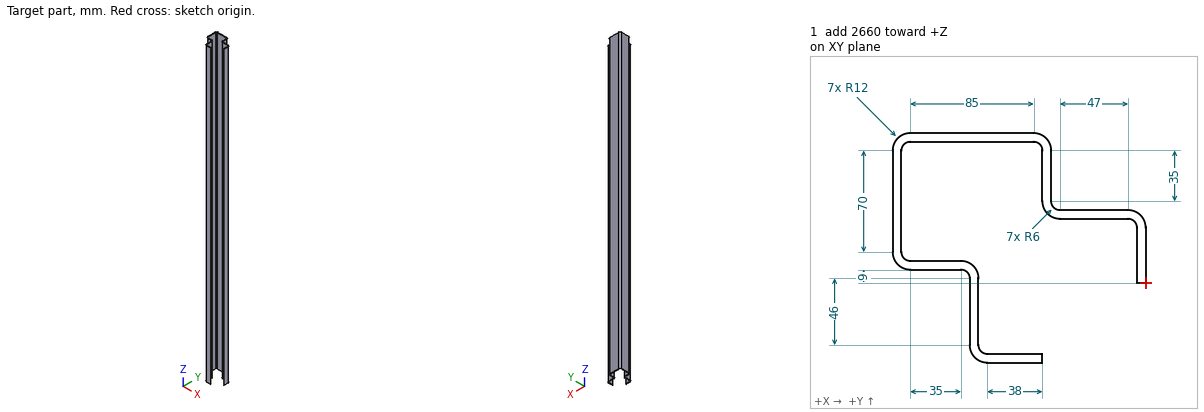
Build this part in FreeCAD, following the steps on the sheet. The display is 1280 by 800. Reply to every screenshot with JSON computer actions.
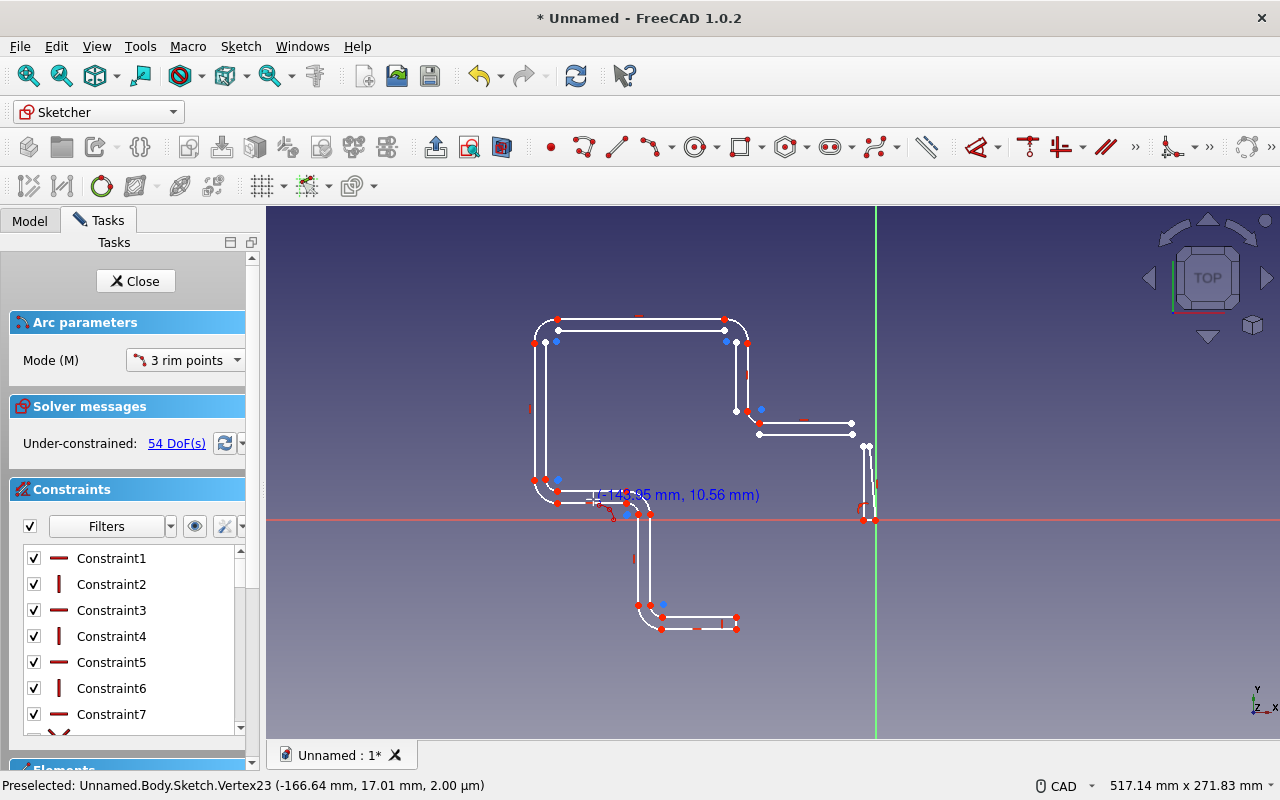
{"action": "scroll", "coordinate": [546, 342], "scroll_direction": "up", "scroll_amount": 2}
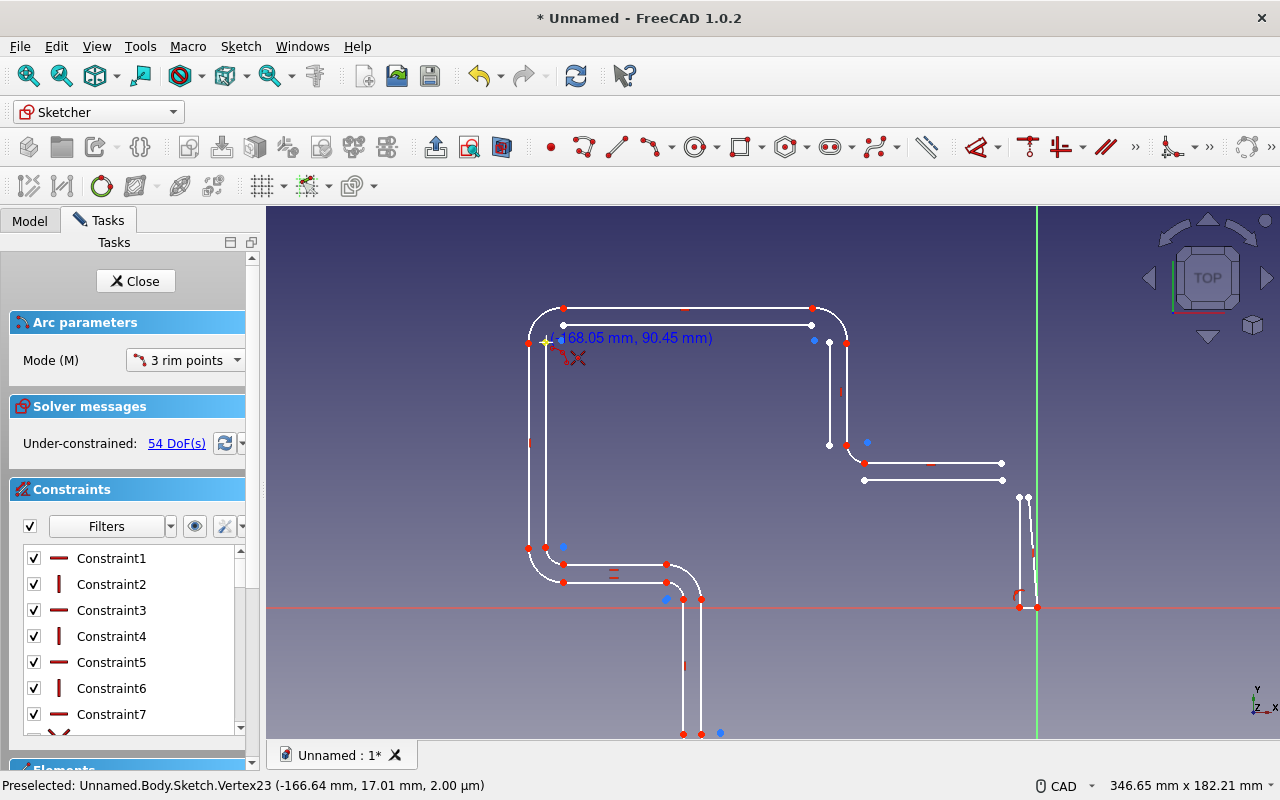
{"action": "left_click", "coordinate": [546, 342]}
{"action": "left_click", "coordinate": [564, 325]}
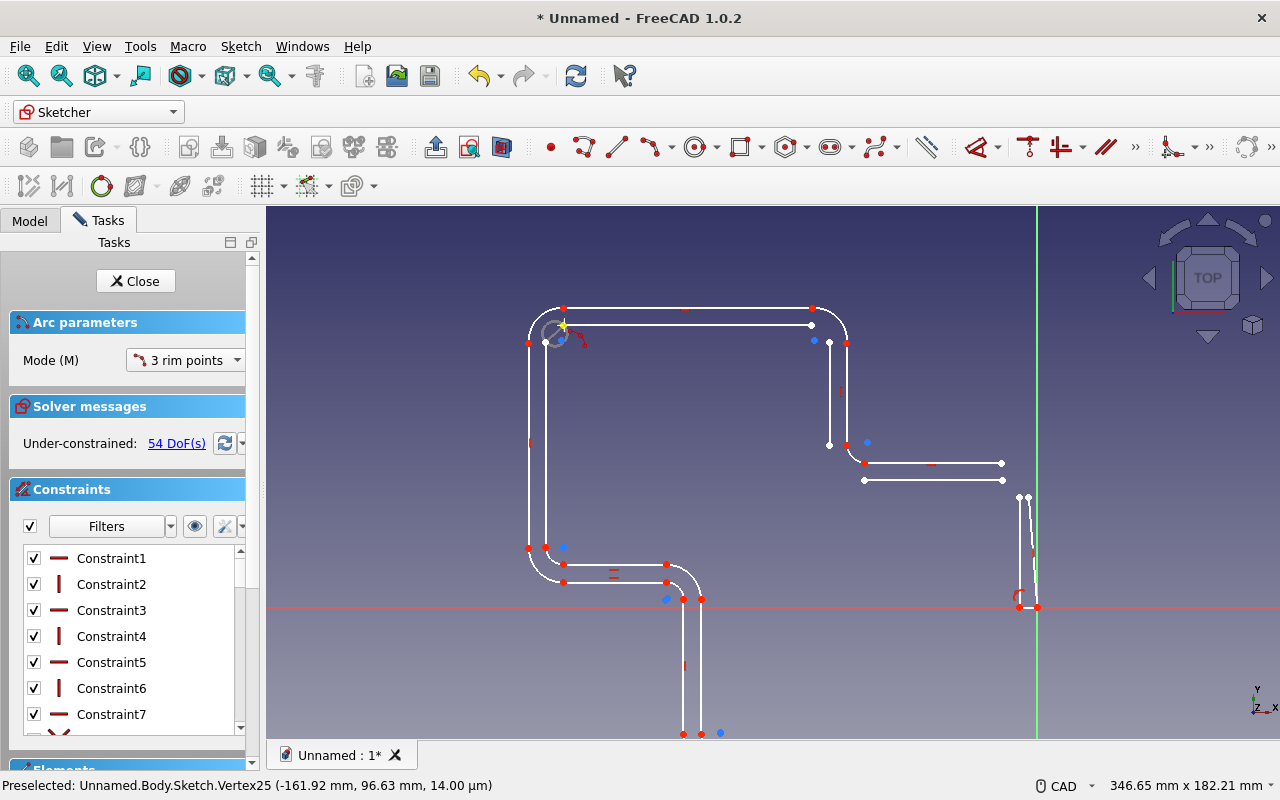
{"action": "scroll", "coordinate": [551, 329], "scroll_direction": "up", "scroll_amount": 6}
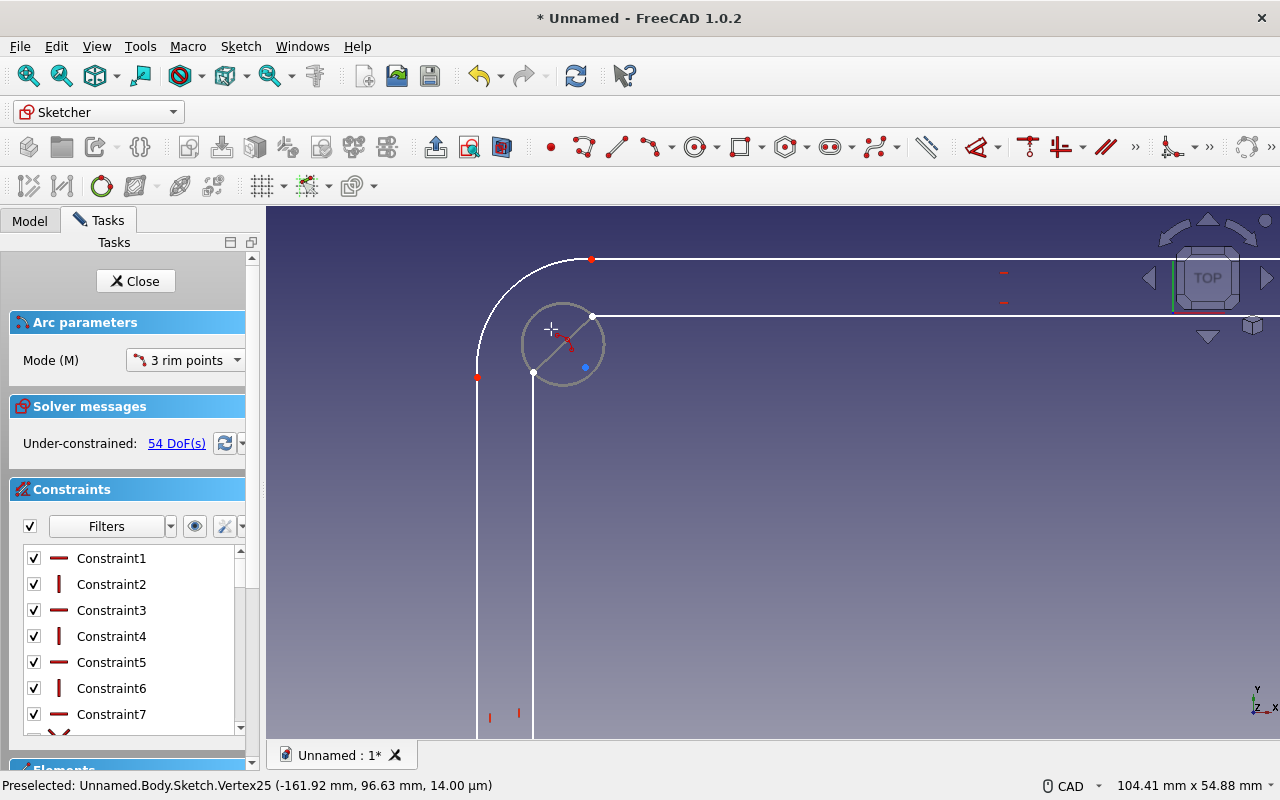
{"action": "left_click", "coordinate": [551, 330]}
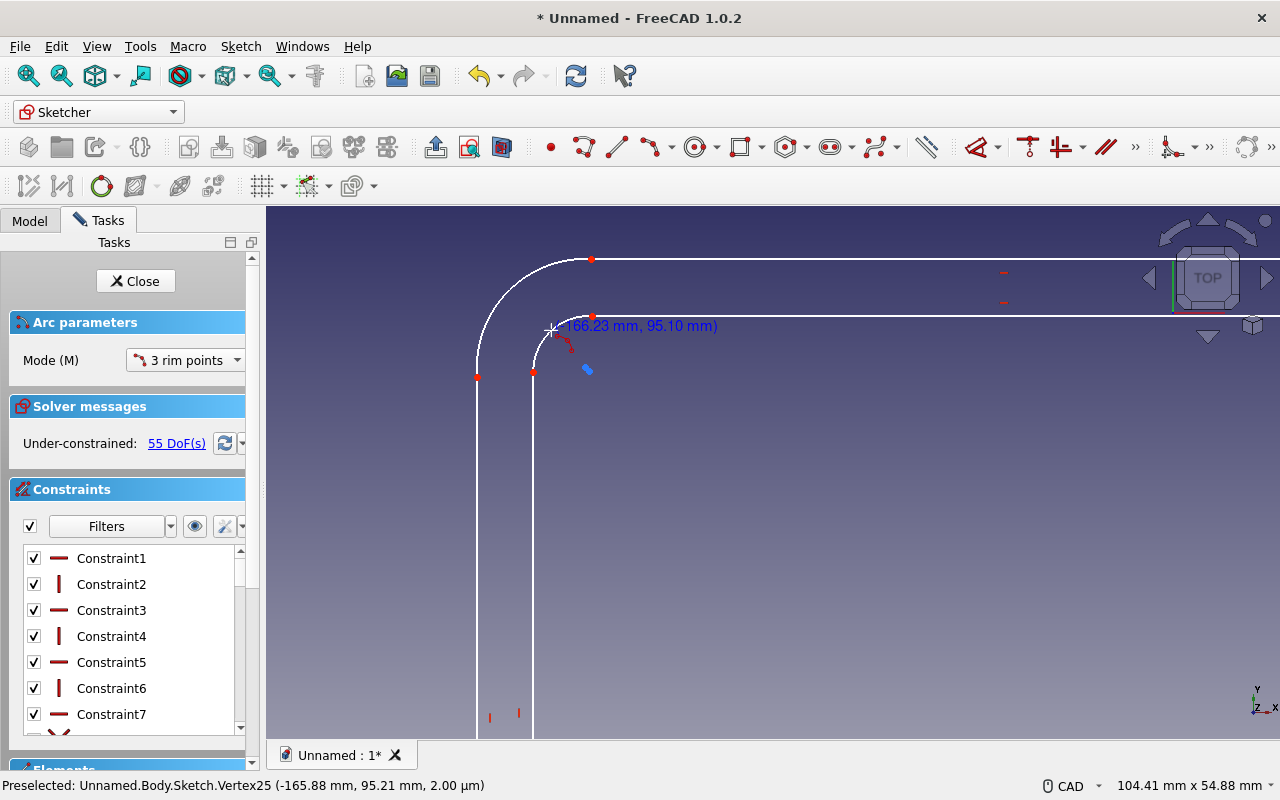
{"action": "scroll", "coordinate": [549, 334], "scroll_direction": "down", "scroll_amount": 8}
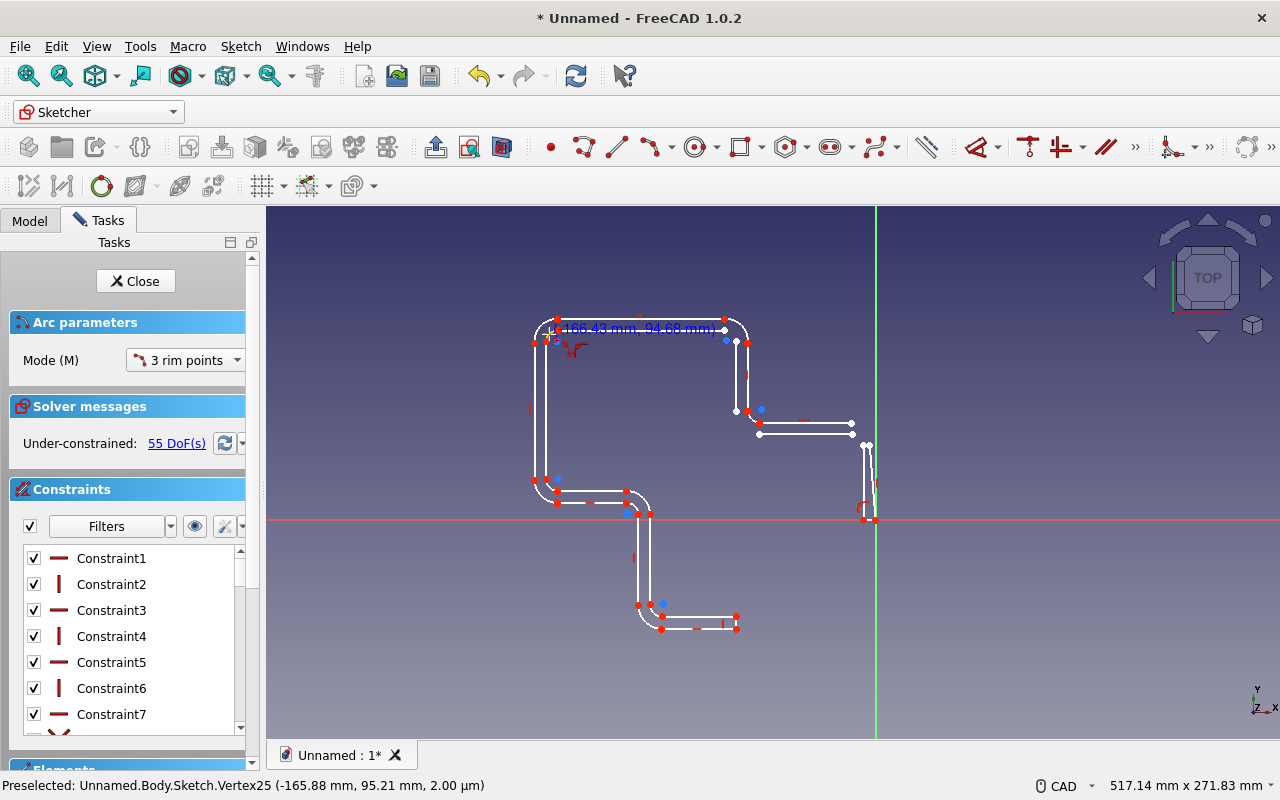
{"action": "scroll", "coordinate": [725, 330], "scroll_direction": "up", "scroll_amount": 2}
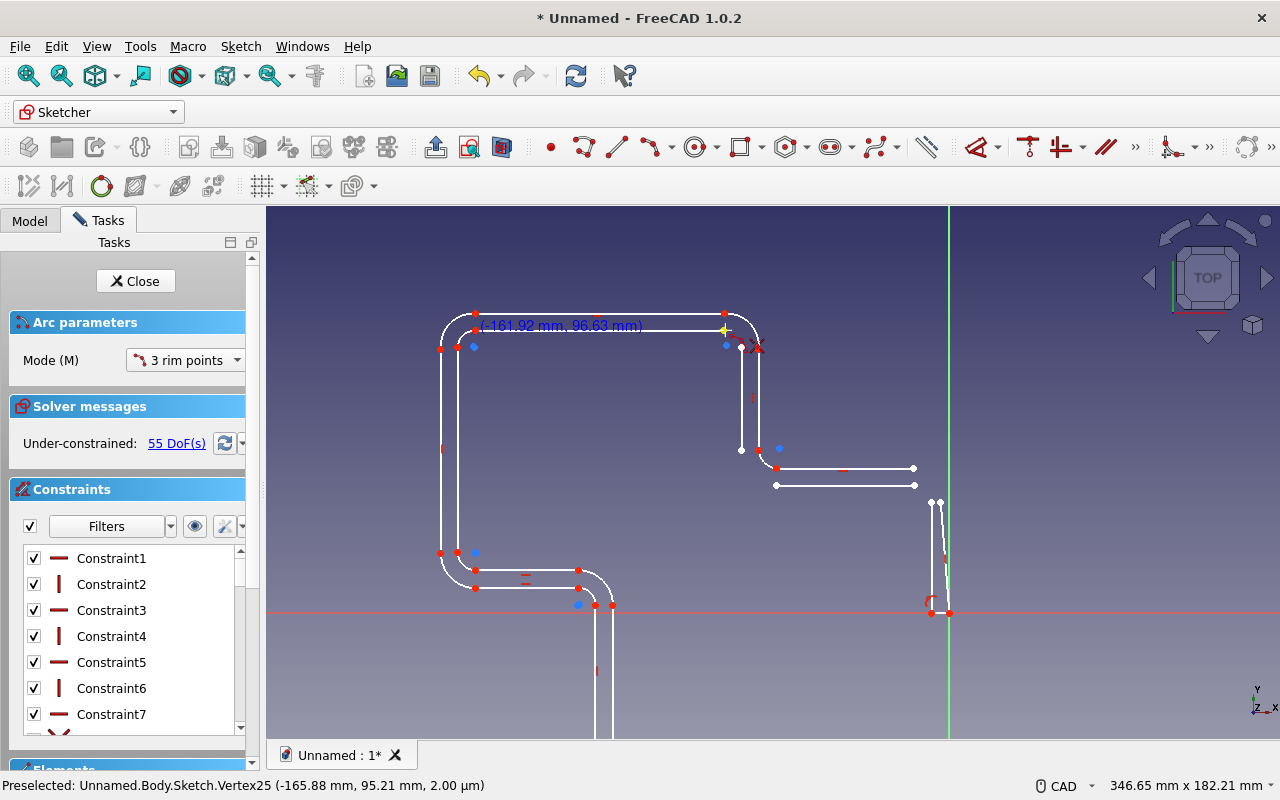
{"action": "left_click", "coordinate": [724, 331]}
{"action": "left_click", "coordinate": [742, 348]}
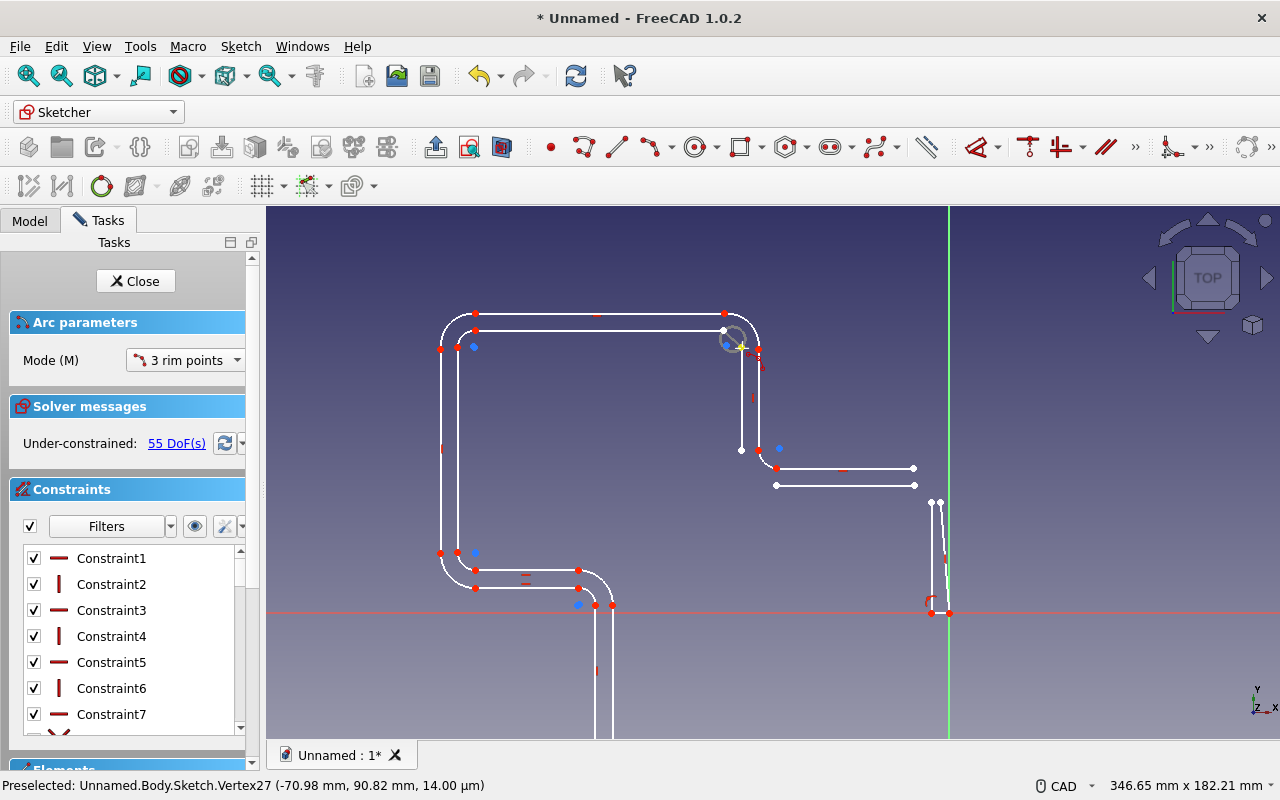
{"action": "scroll", "coordinate": [737, 335], "scroll_direction": "up", "scroll_amount": 6}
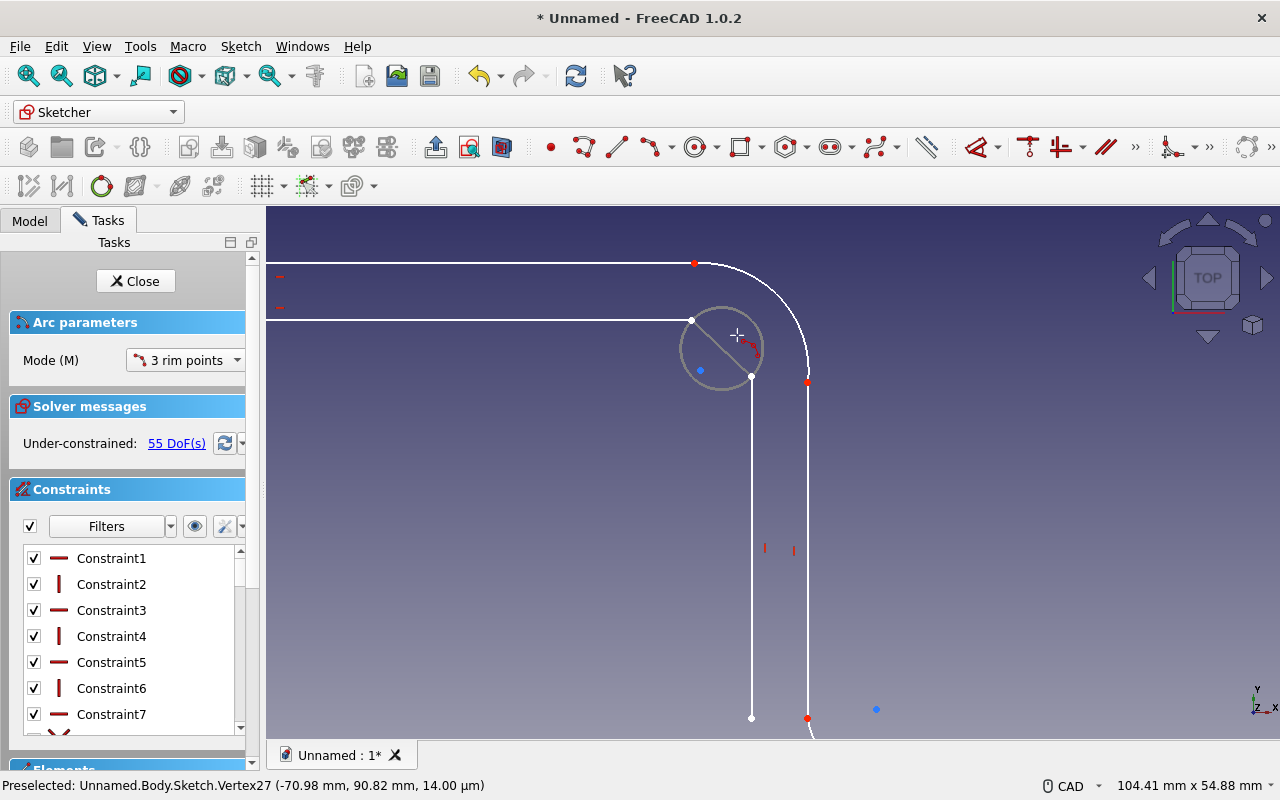
{"action": "left_click", "coordinate": [734, 334]}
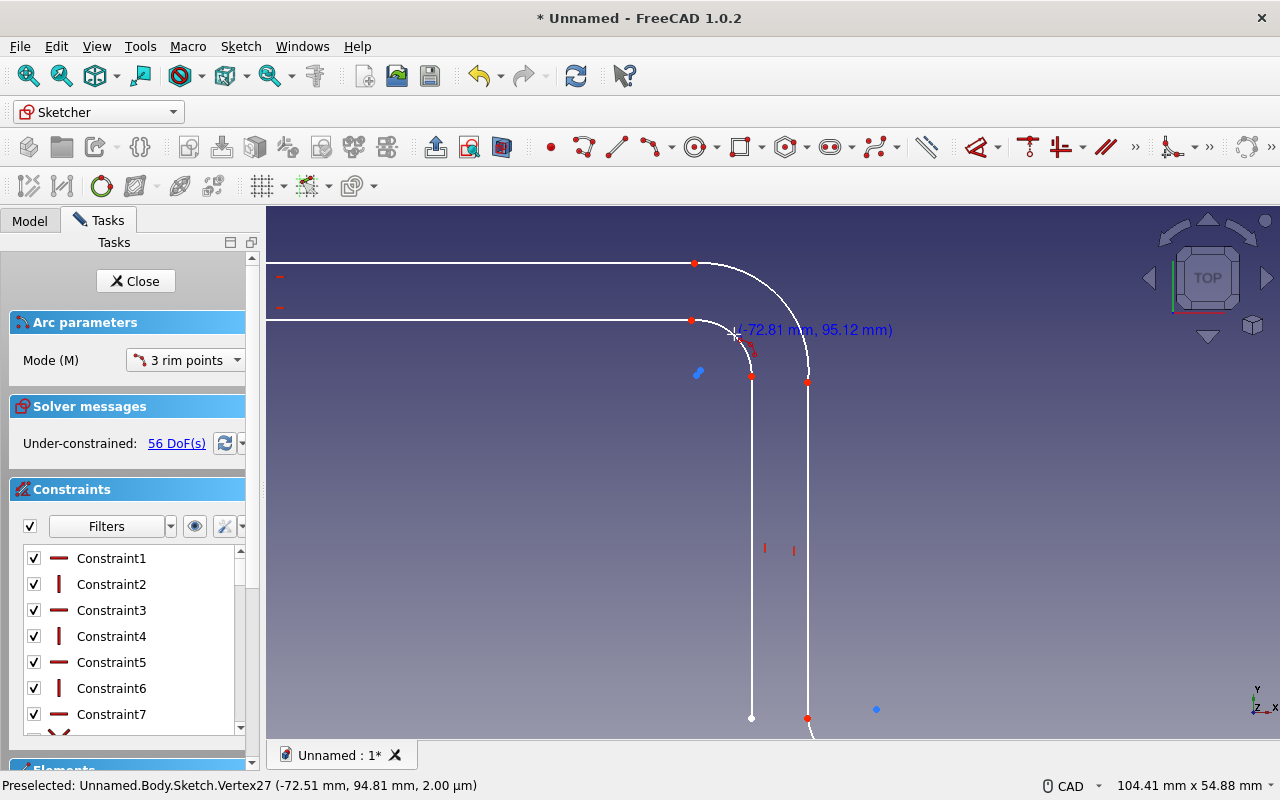
{"action": "scroll", "coordinate": [732, 333], "scroll_direction": "down", "scroll_amount": 8}